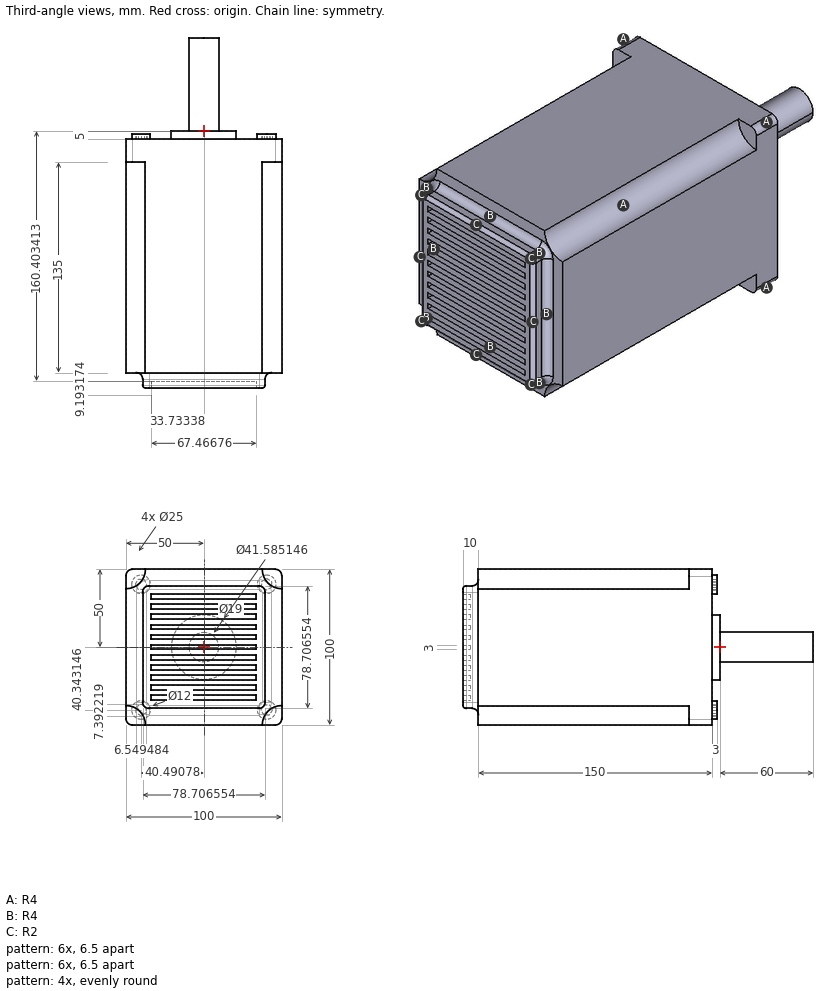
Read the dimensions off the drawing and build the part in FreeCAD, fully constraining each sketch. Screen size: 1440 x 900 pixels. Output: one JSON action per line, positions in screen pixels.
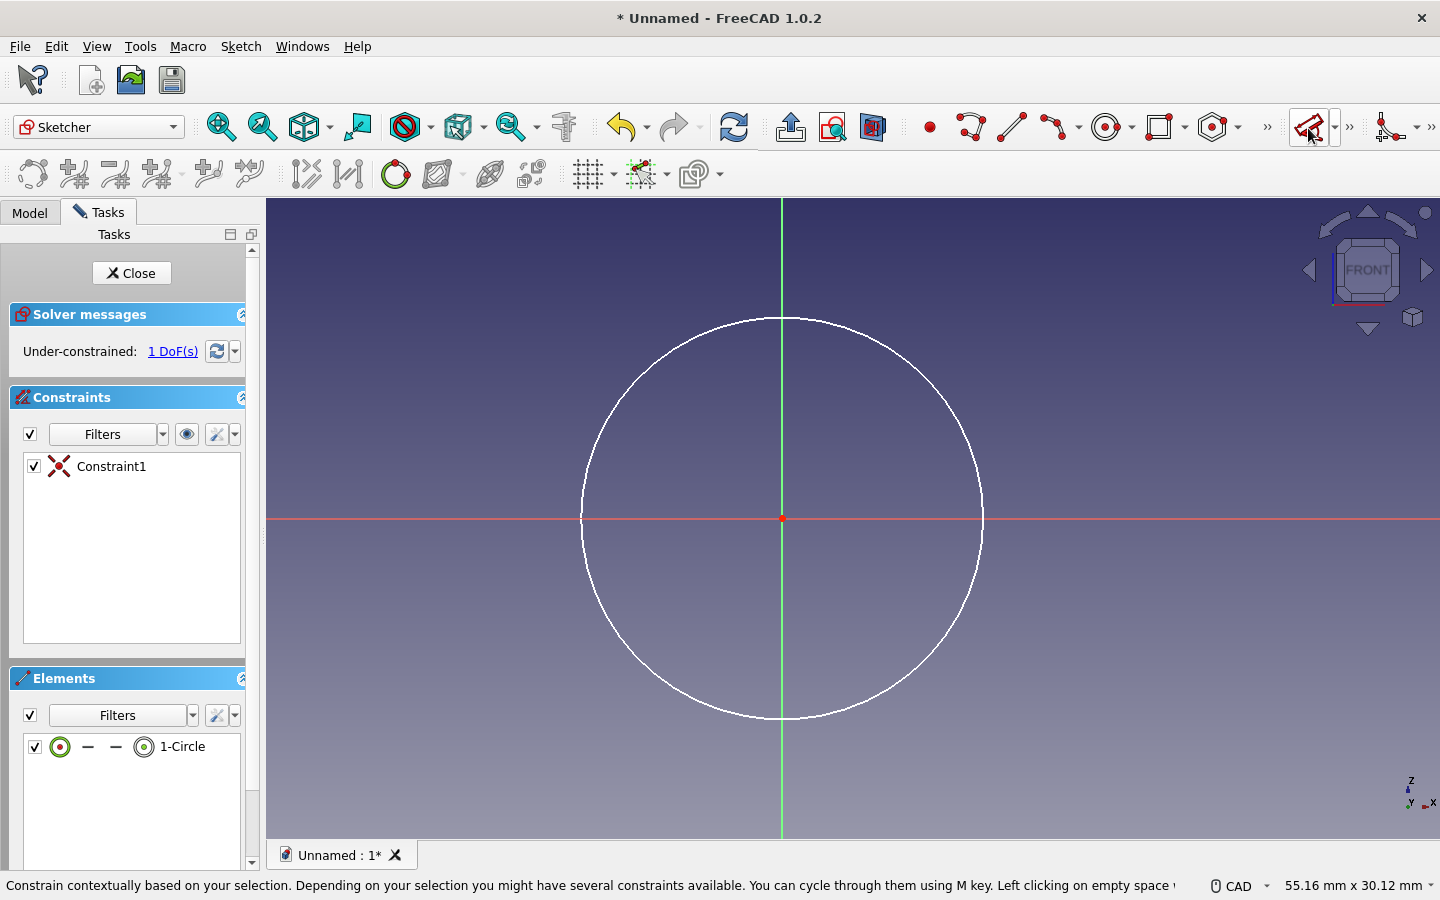
{"action": "left_click", "coordinate": [924, 376]}
{"action": "left_click", "coordinate": [947, 353]}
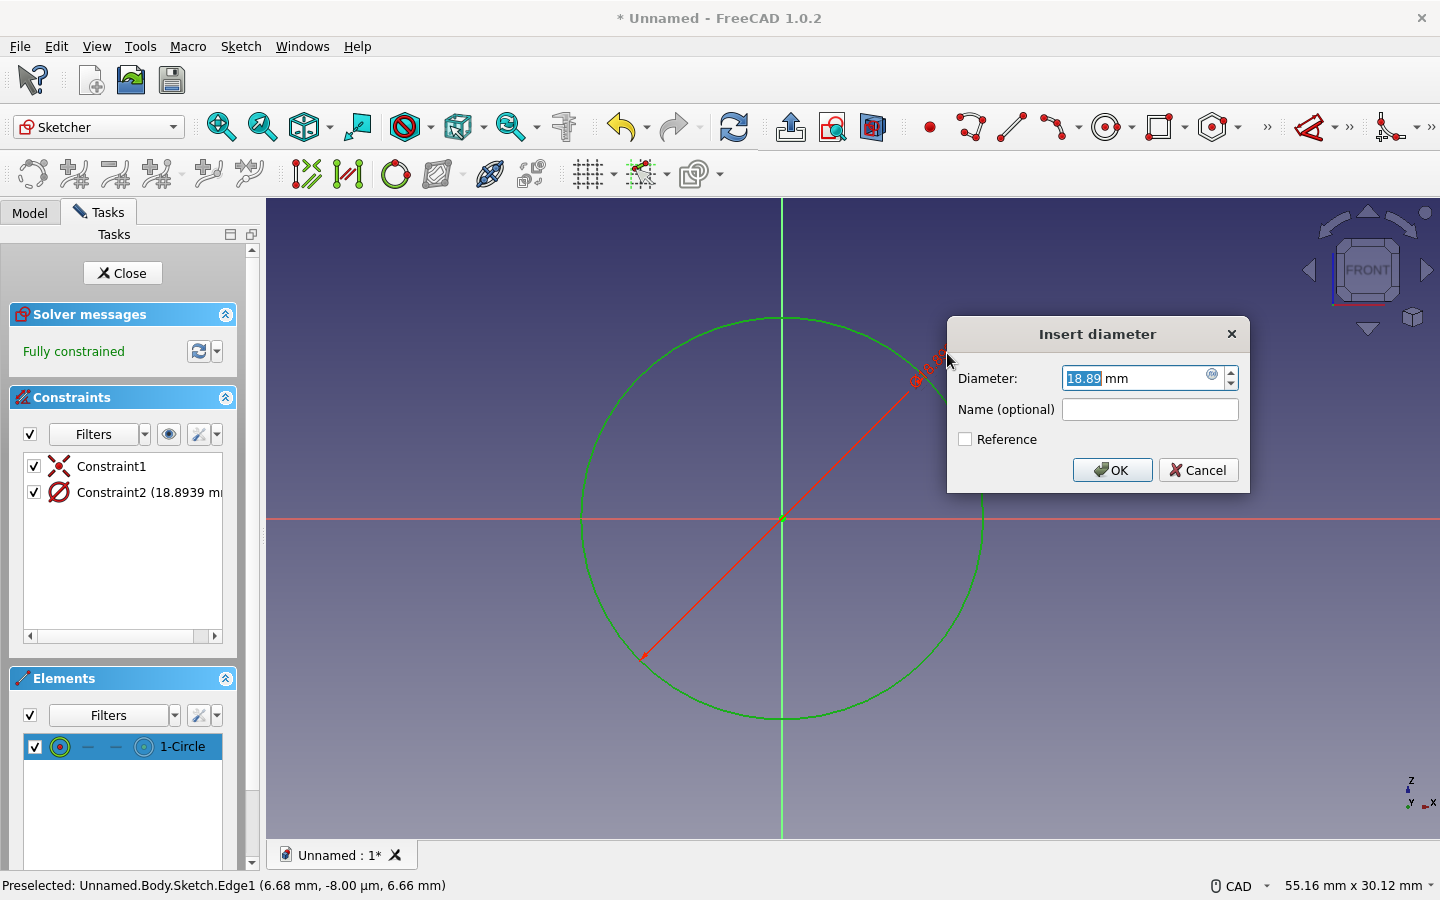
{"action": "type", "text": "19"}
{"action": "key", "text": "Return"}
{"action": "key", "text": "Escape"}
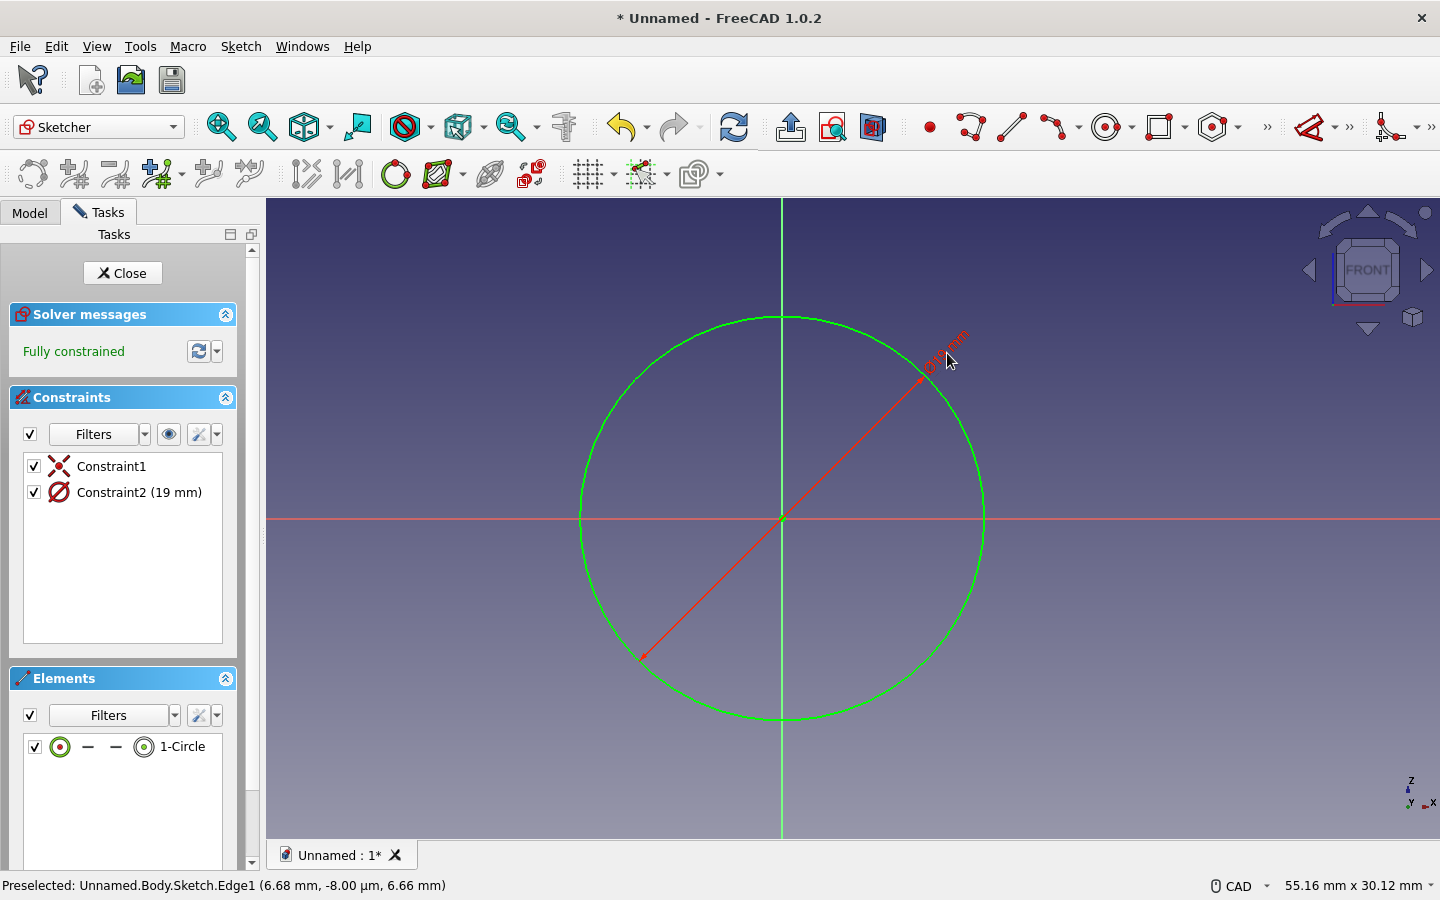
{"action": "left_click", "coordinate": [123, 273]}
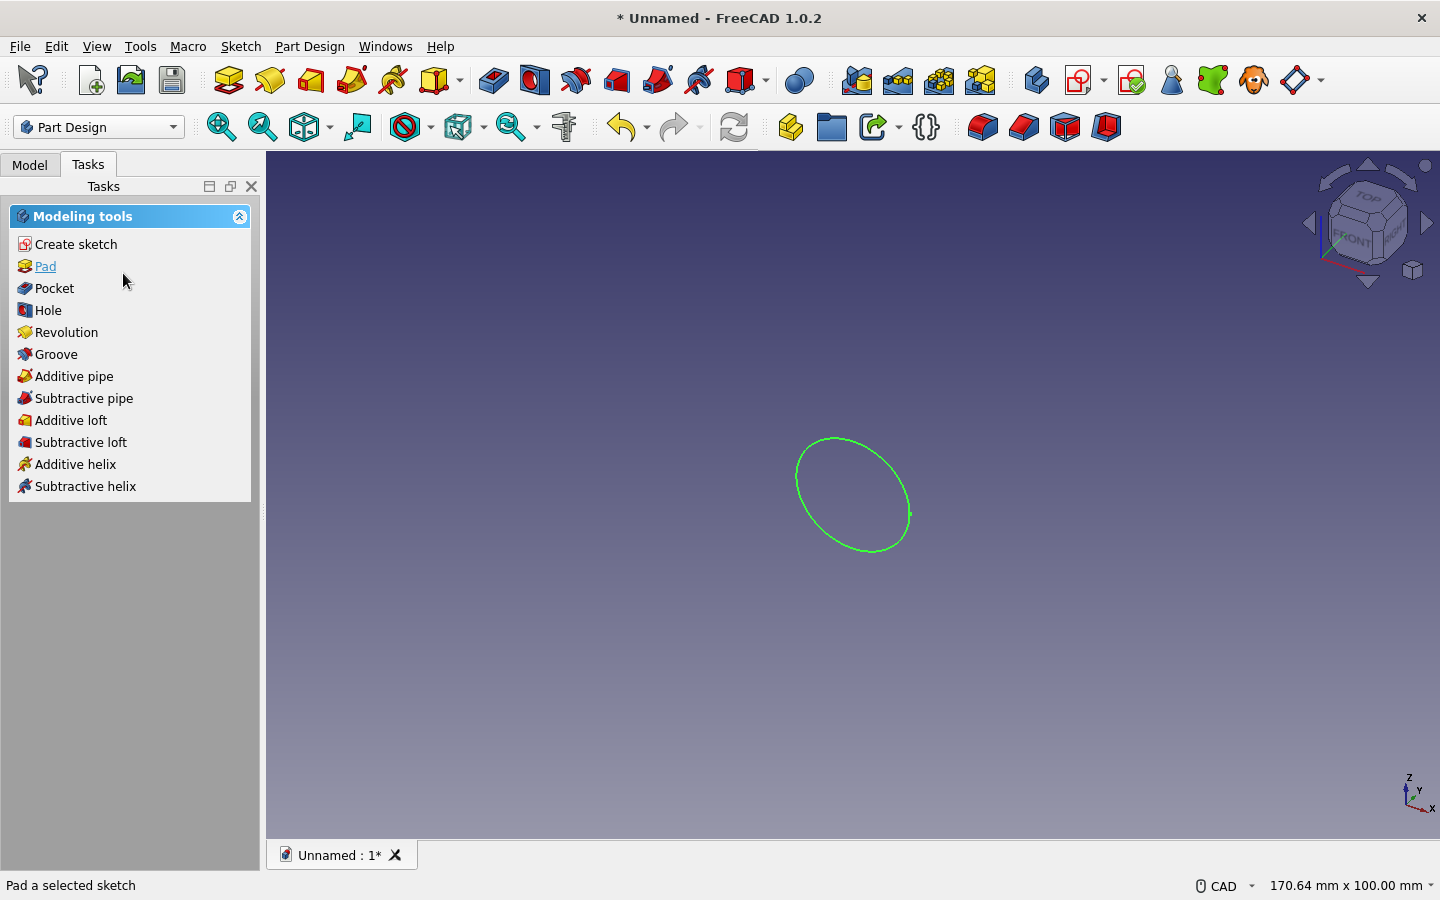
{"action": "left_click", "coordinate": [229, 80]}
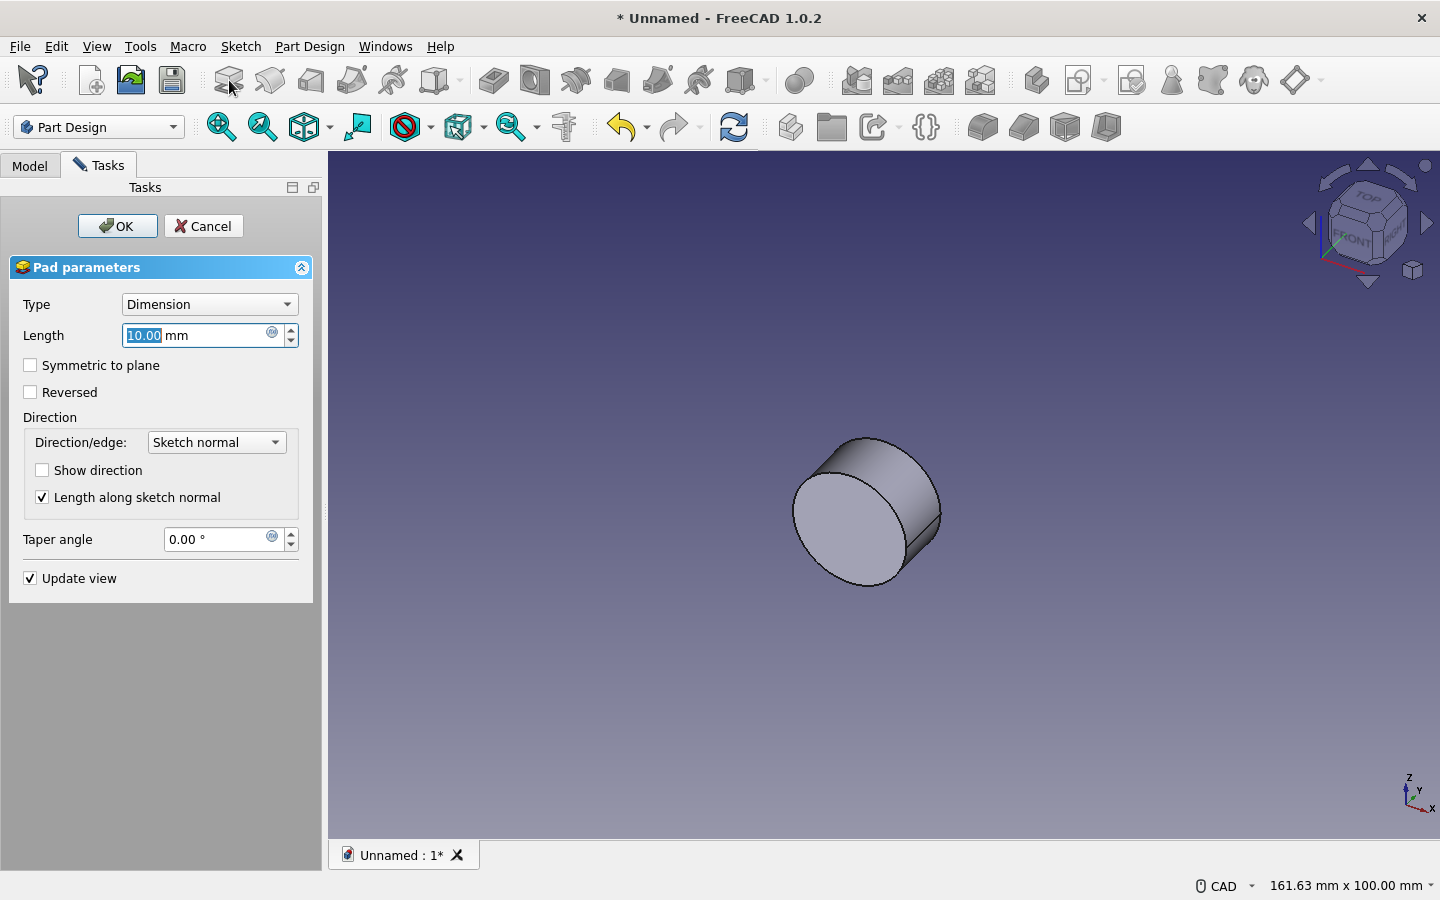
{"action": "type", "text": "60"}
{"action": "key", "text": "Tab"}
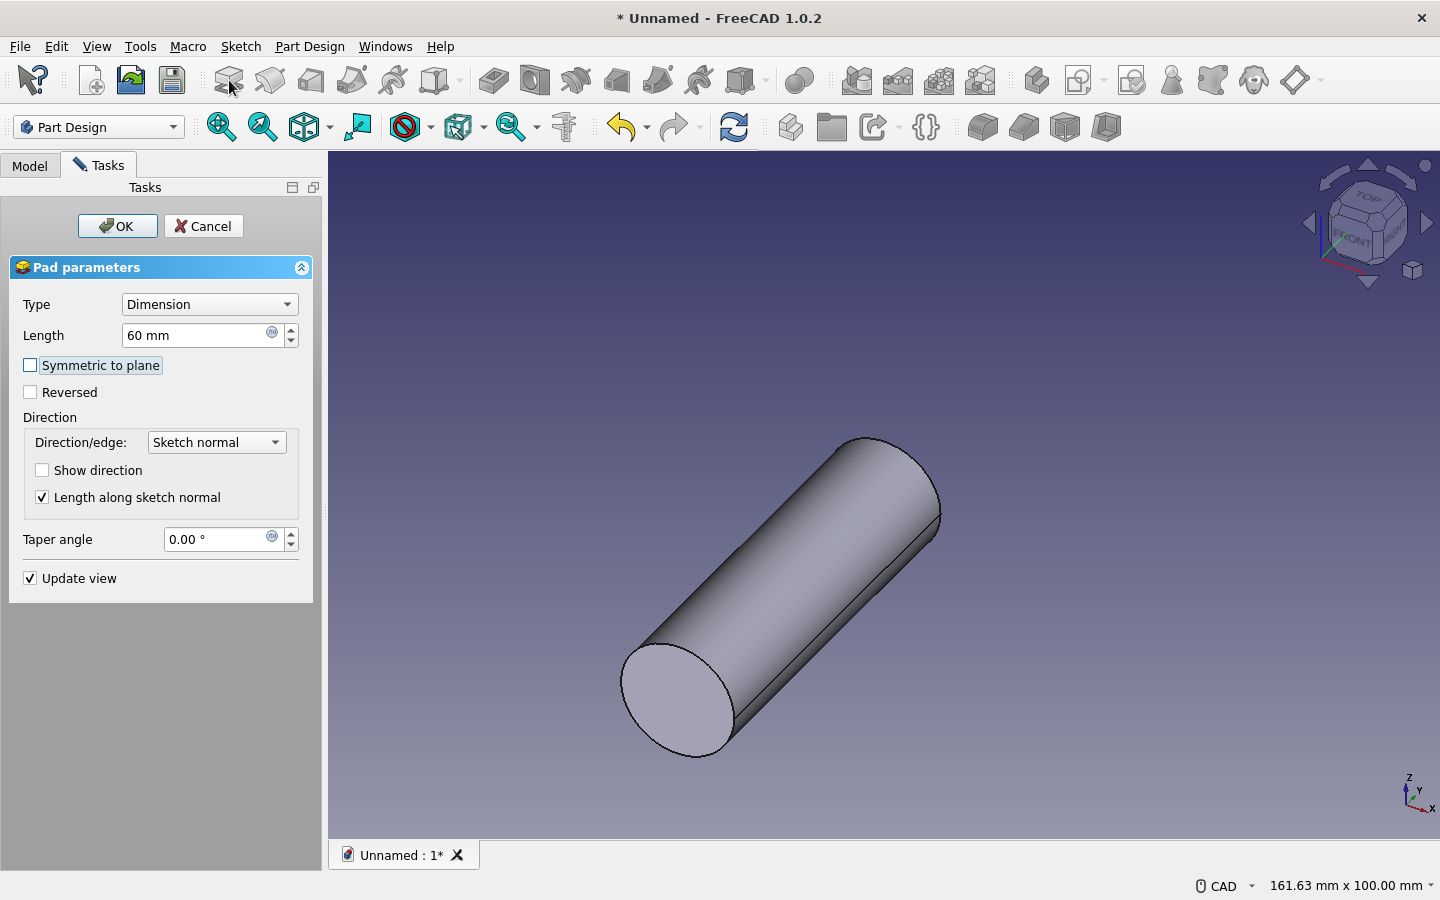
{"action": "left_click", "coordinate": [31, 392]}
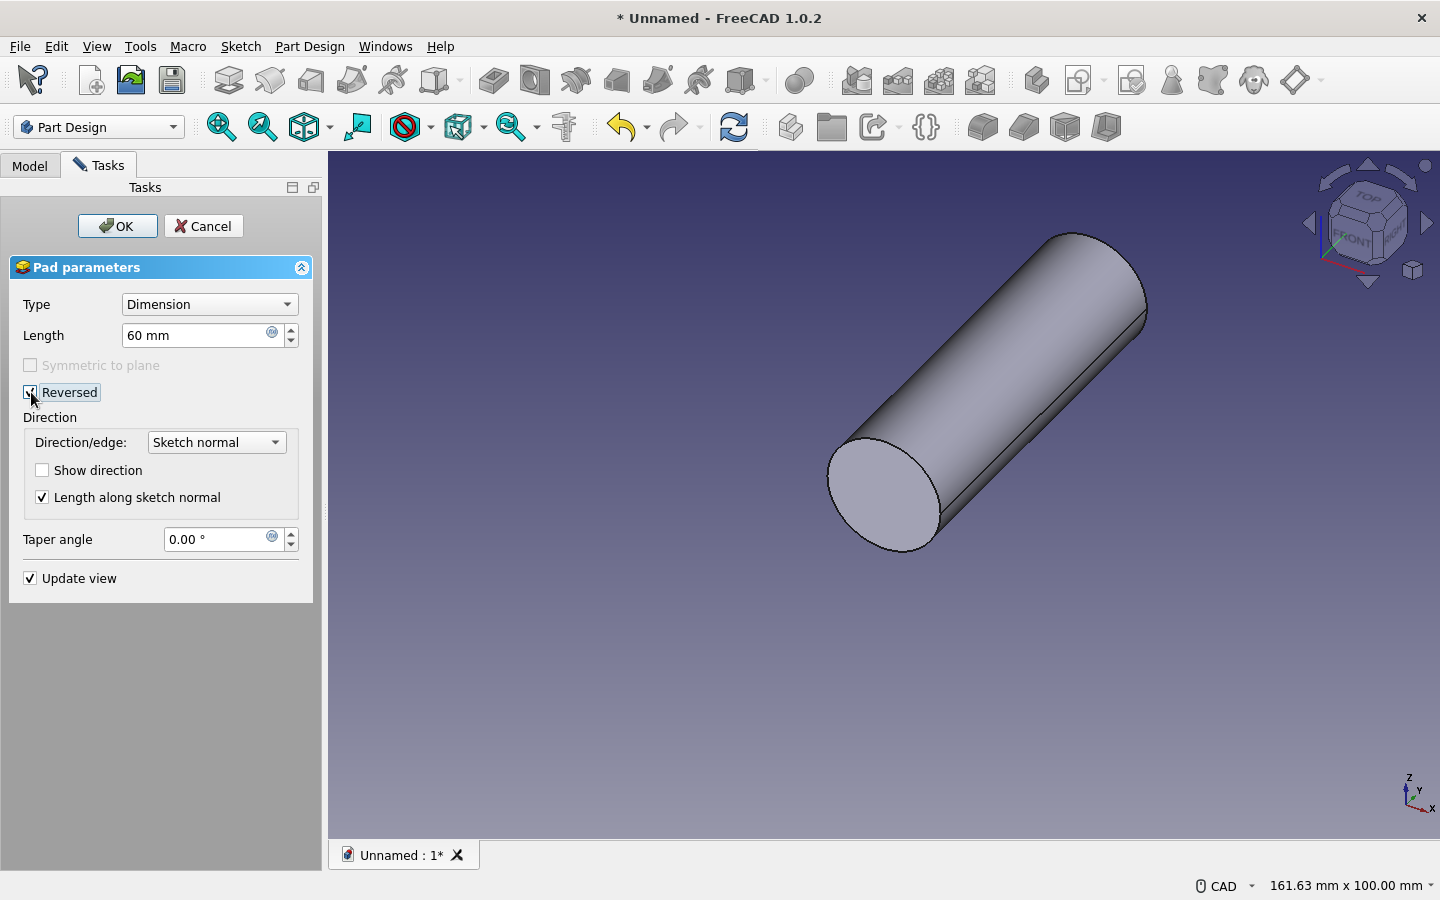
{"action": "left_click", "coordinate": [118, 226]}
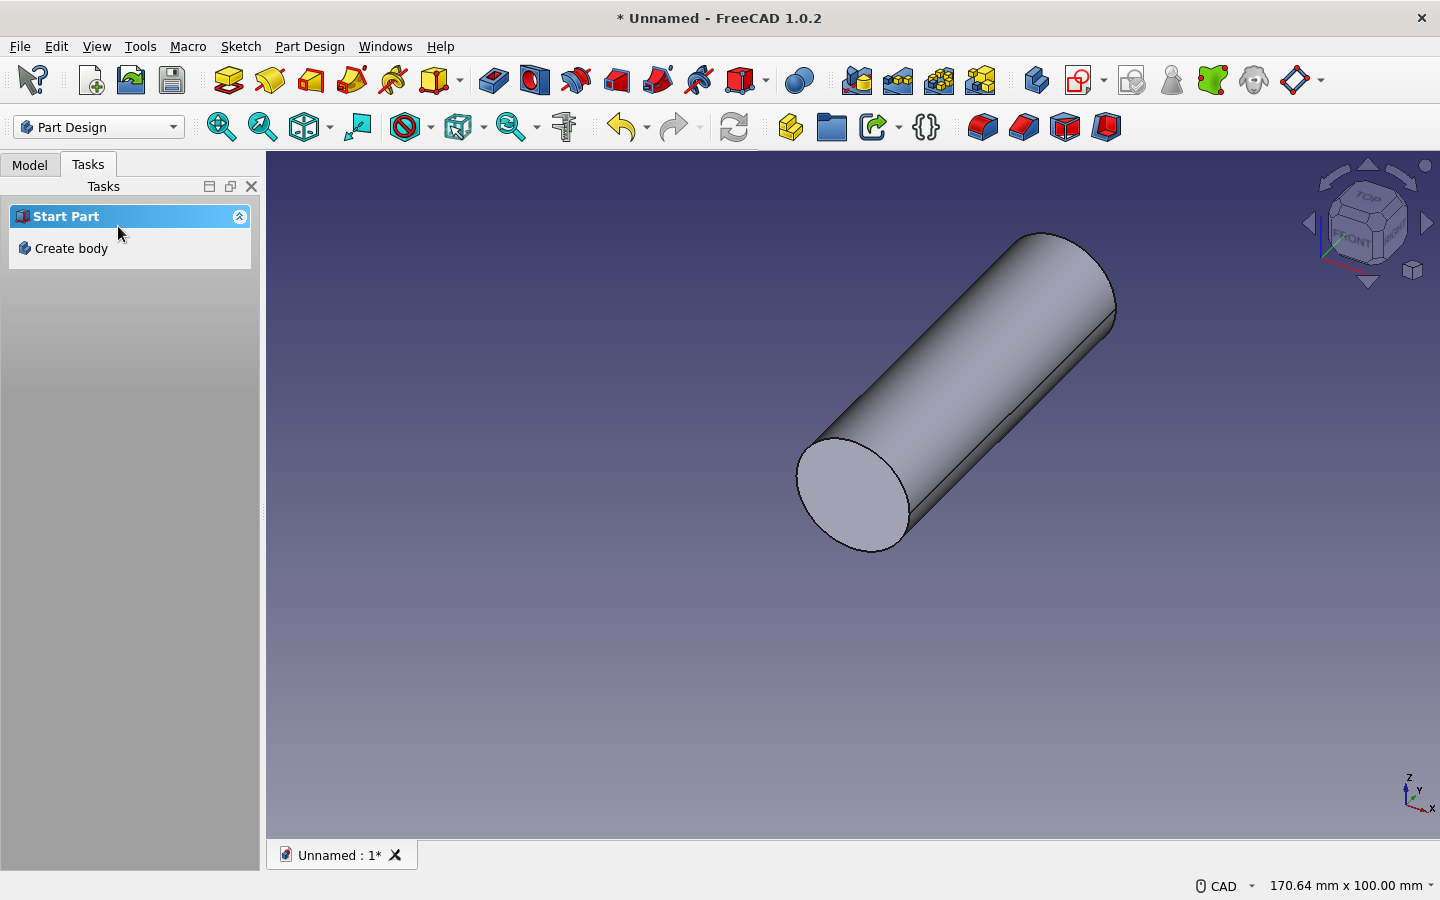
{"action": "left_click", "coordinate": [1078, 80]}